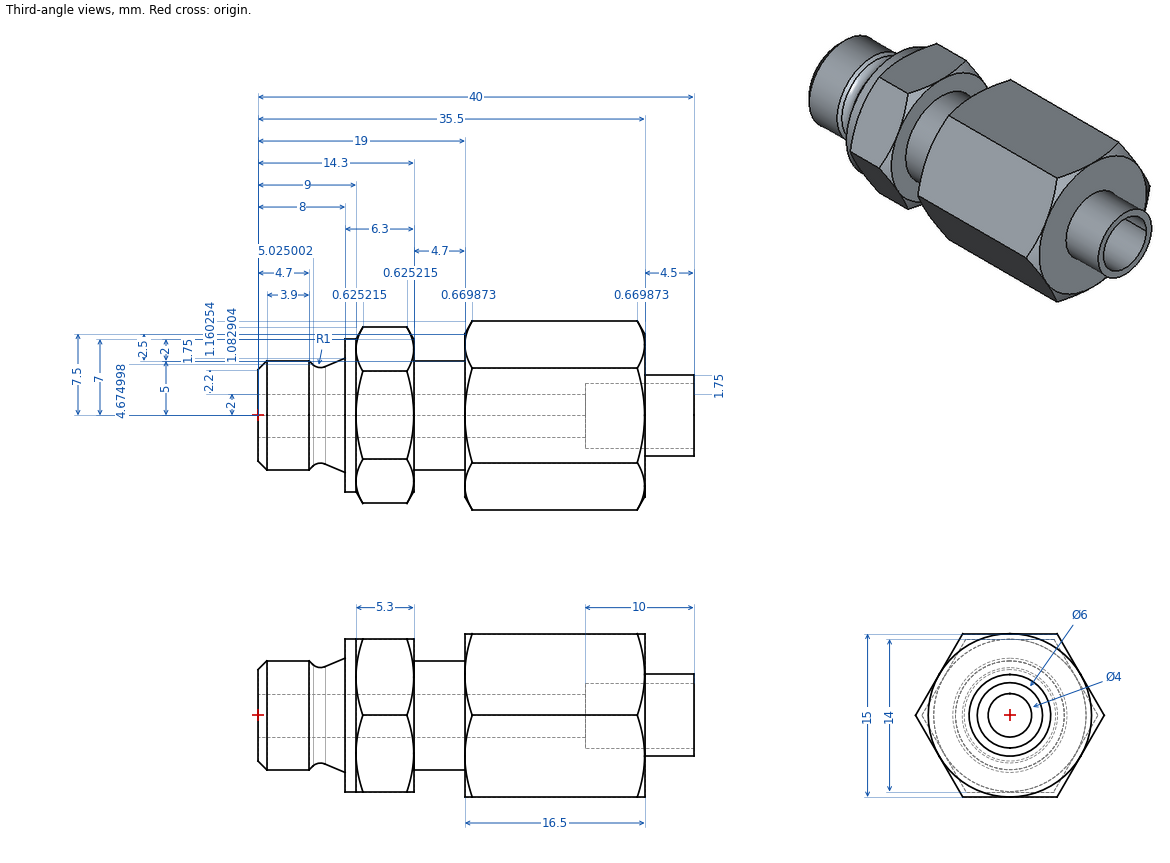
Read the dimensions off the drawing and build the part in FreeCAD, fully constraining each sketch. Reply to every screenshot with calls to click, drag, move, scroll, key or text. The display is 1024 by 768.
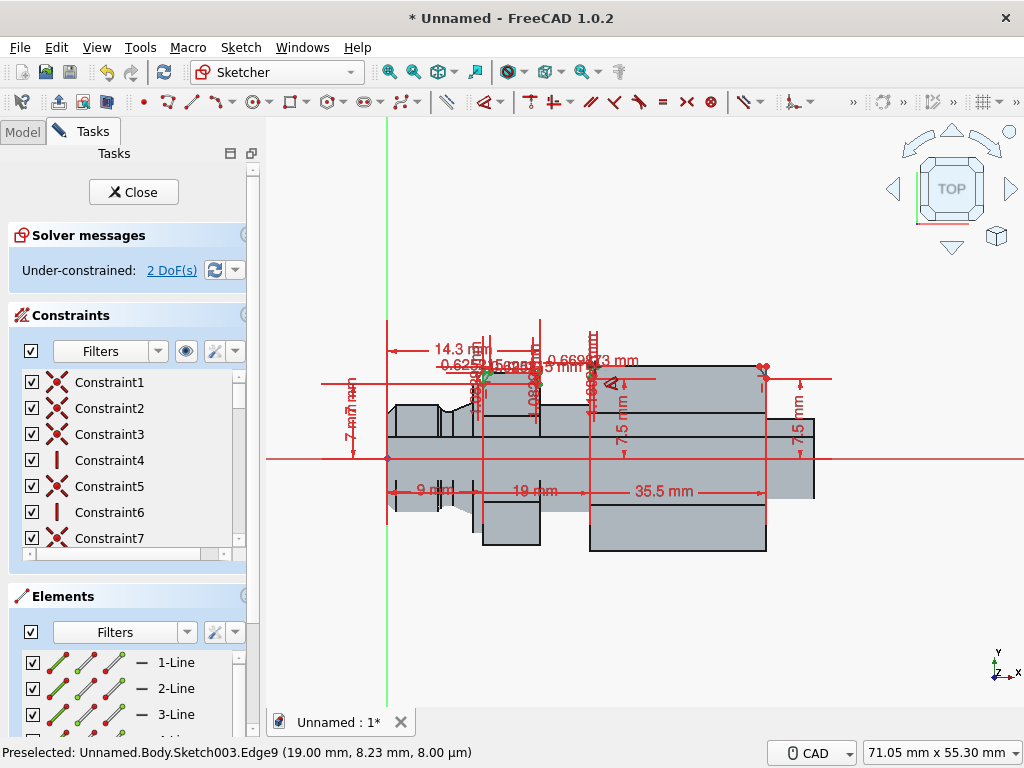
scroll(766, 375, up, 11)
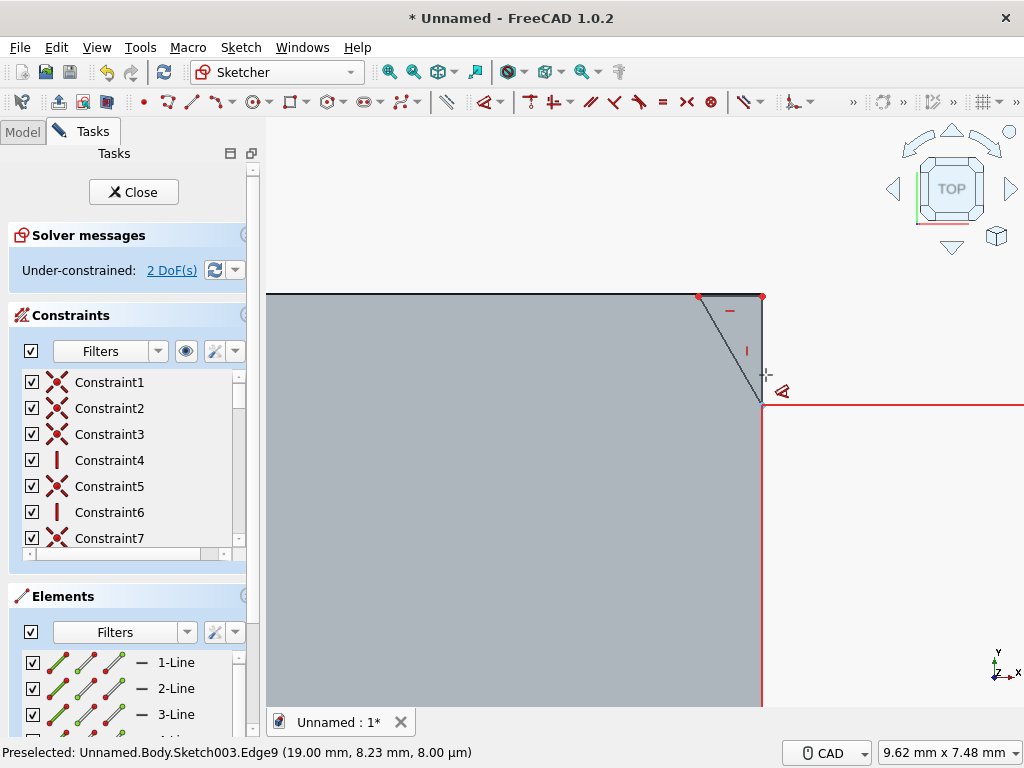
click(762, 373)
click(796, 351)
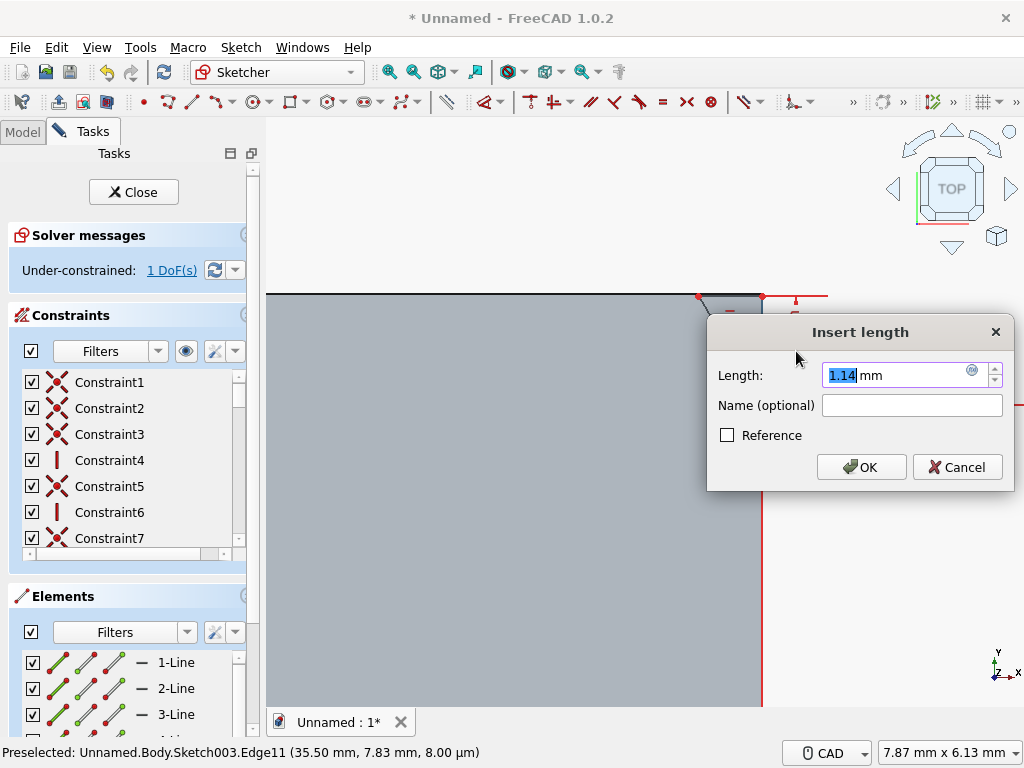
text(1.160254)
key(Return)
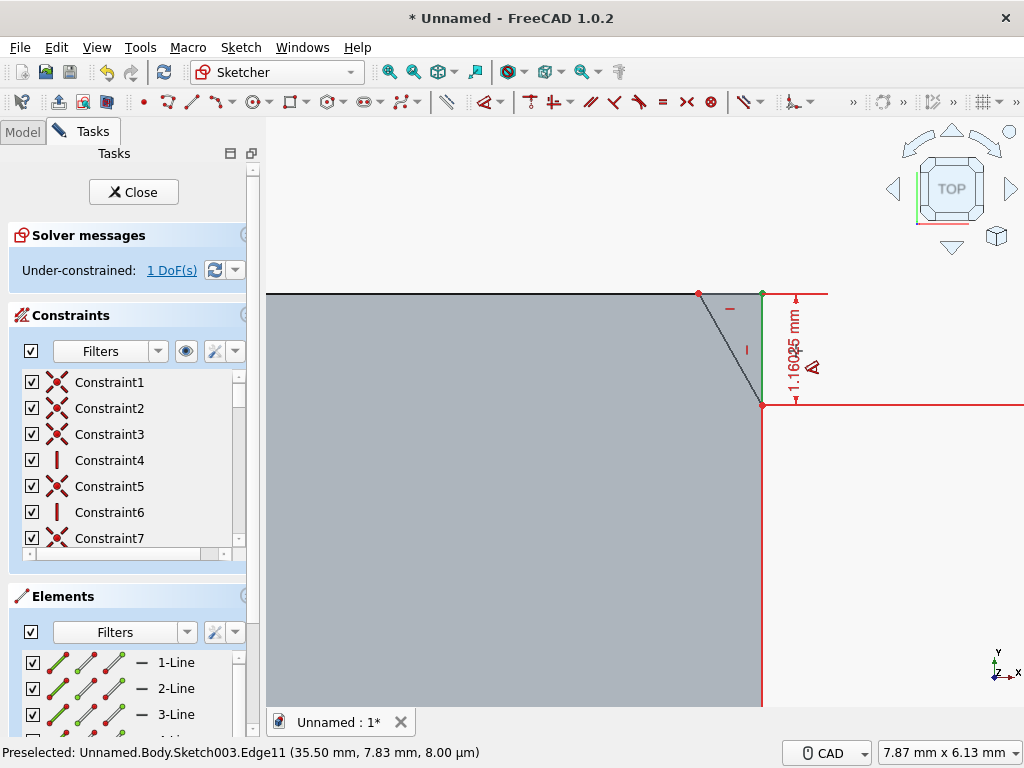
click(743, 294)
click(730, 260)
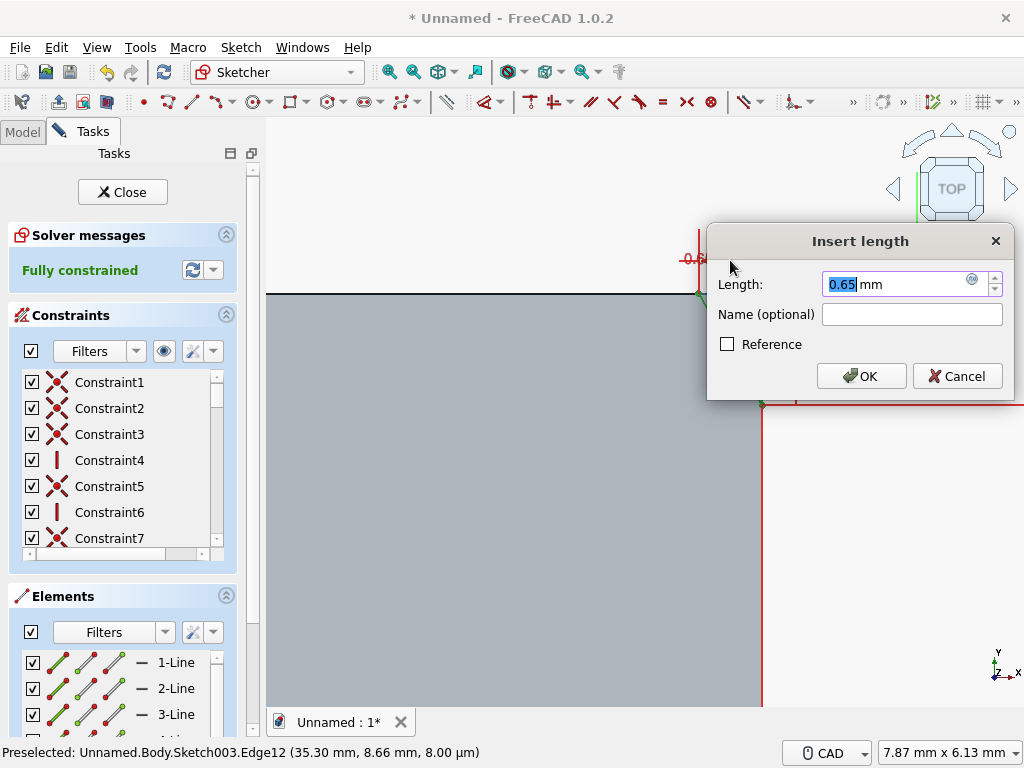
text(0.669873)
key(Return)
key(Escape)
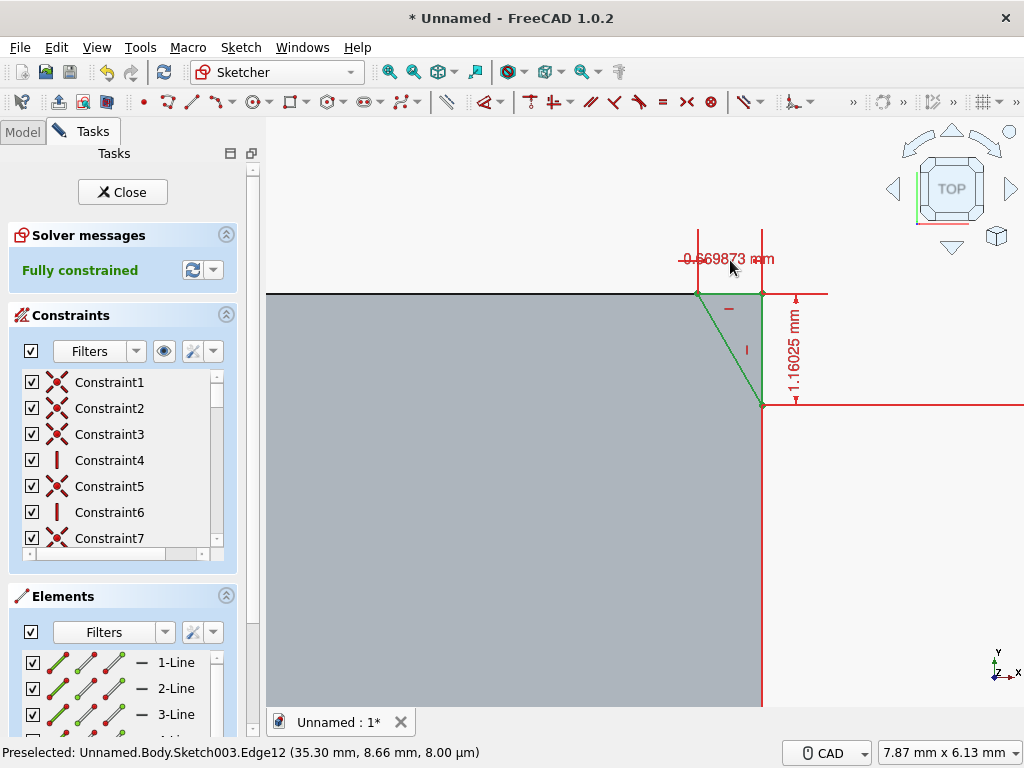
click(123, 192)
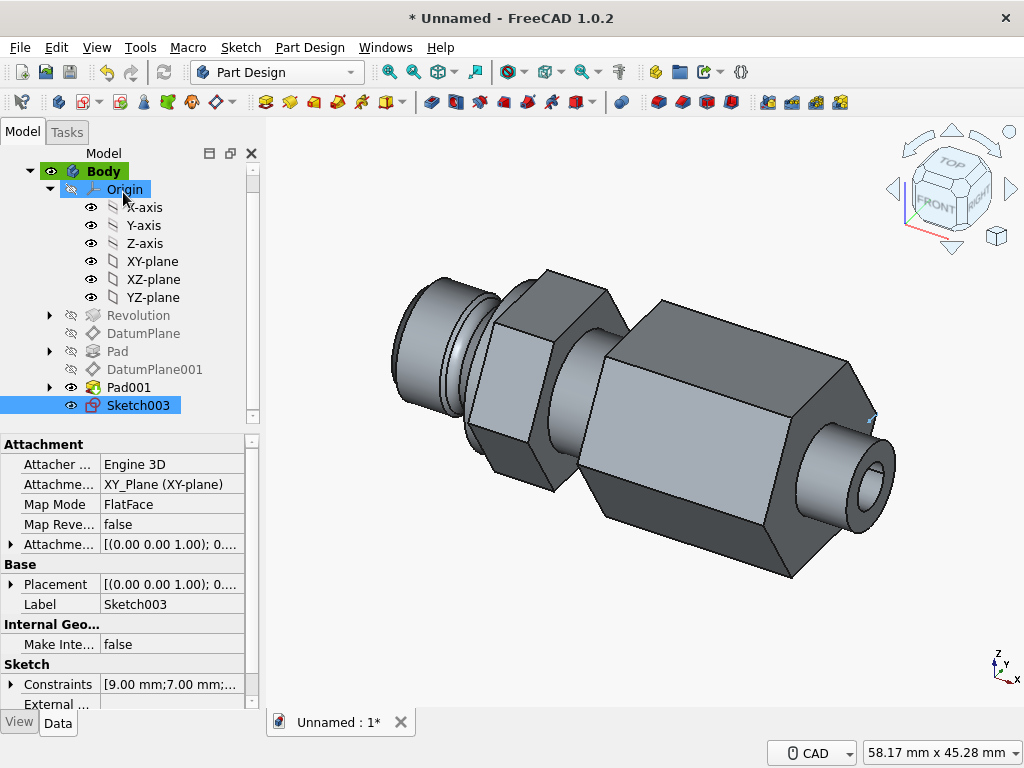
click(480, 102)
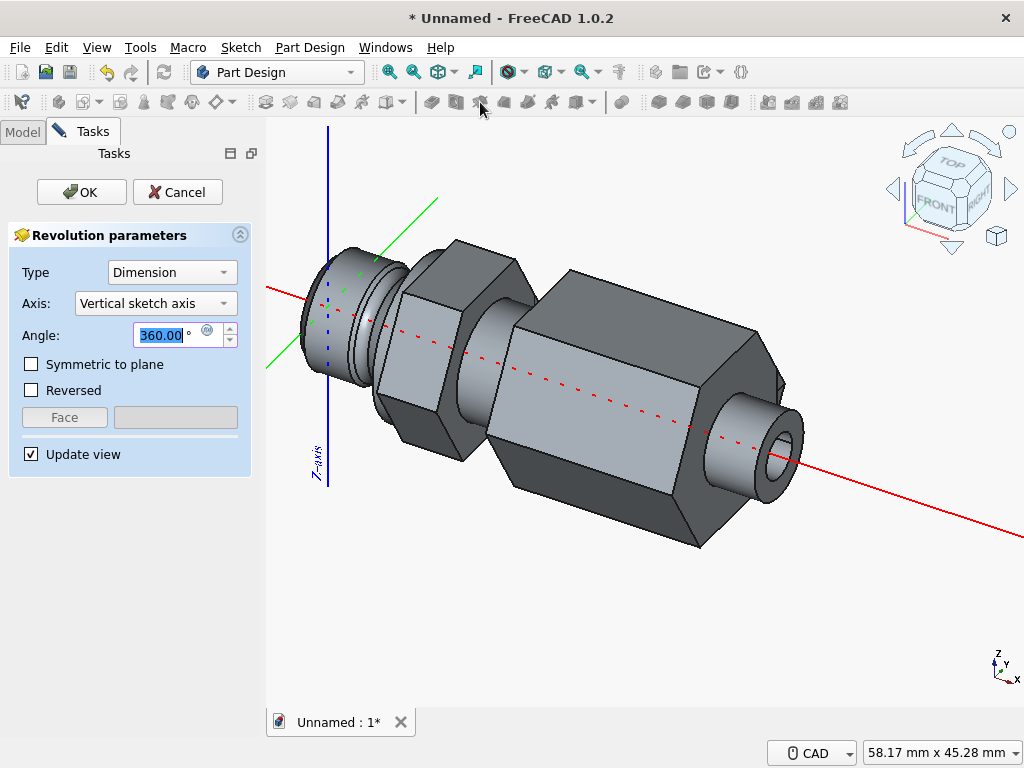
click(156, 304)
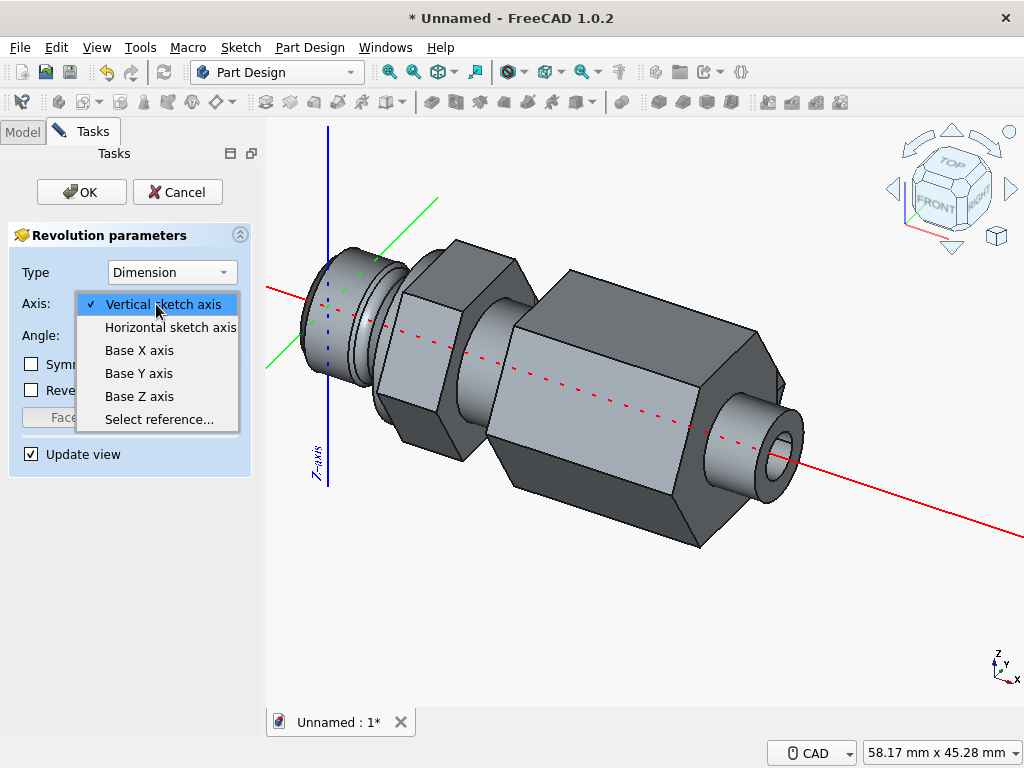
click(156, 328)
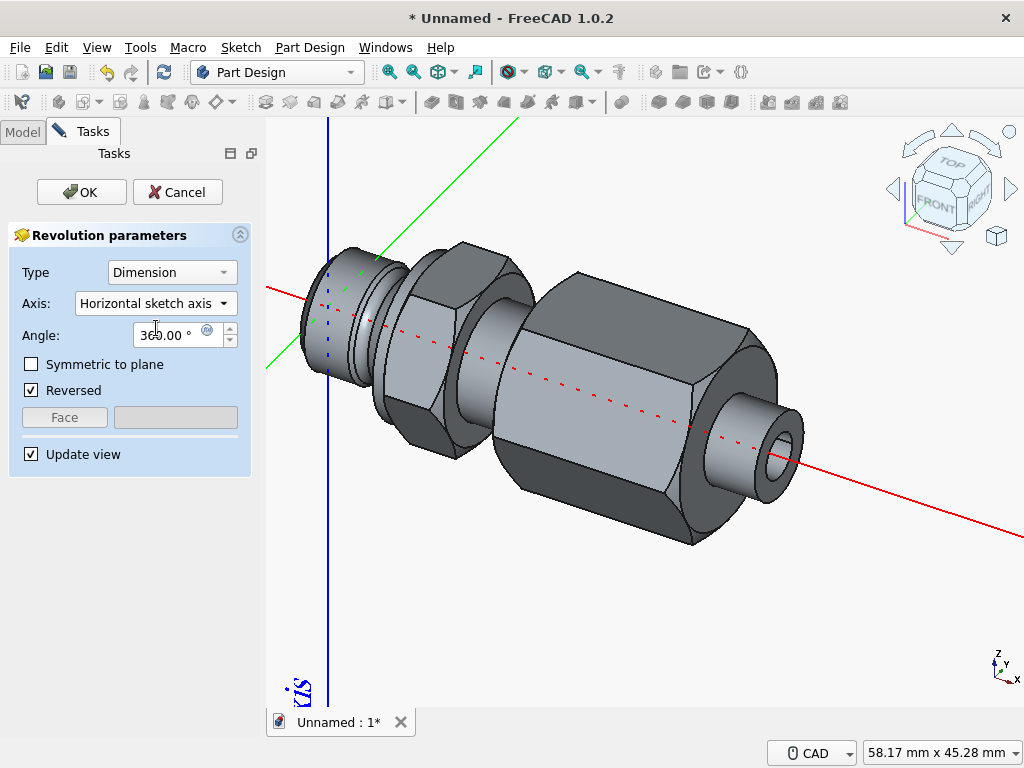
click(82, 192)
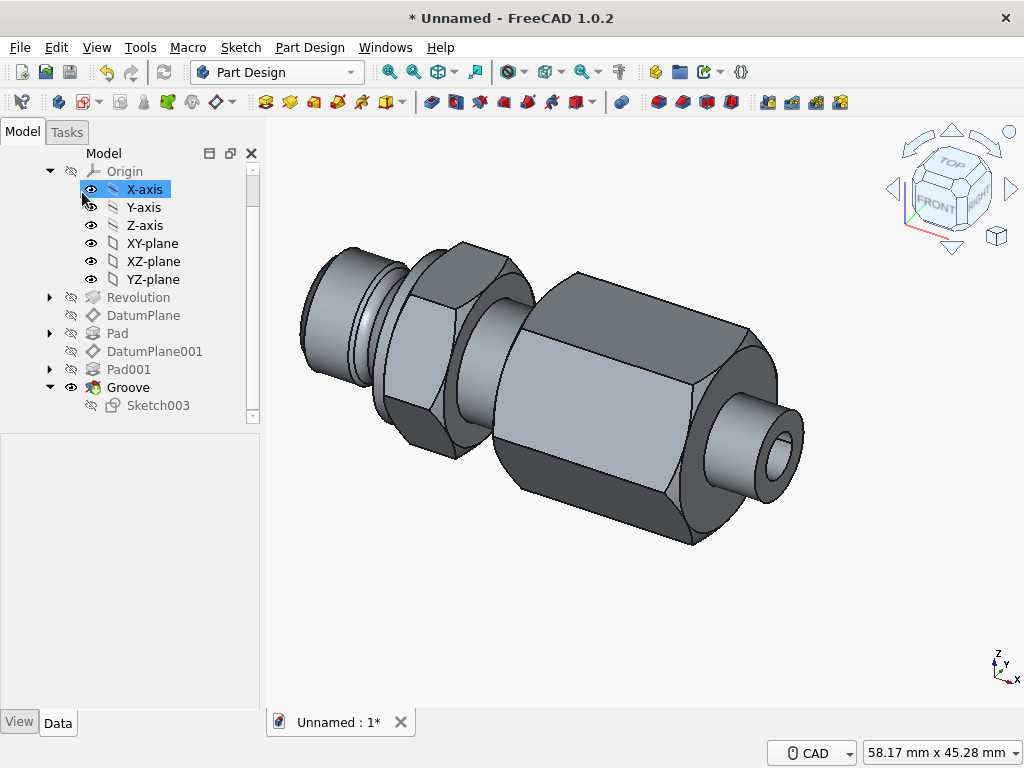
click(793, 419)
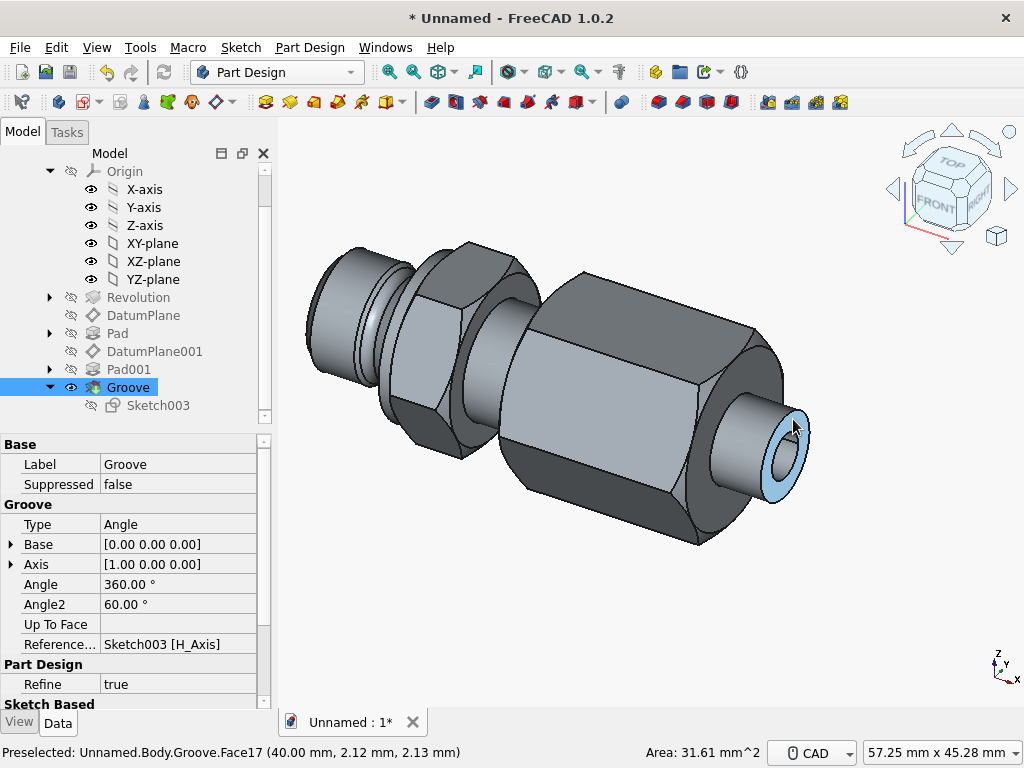
click(84, 102)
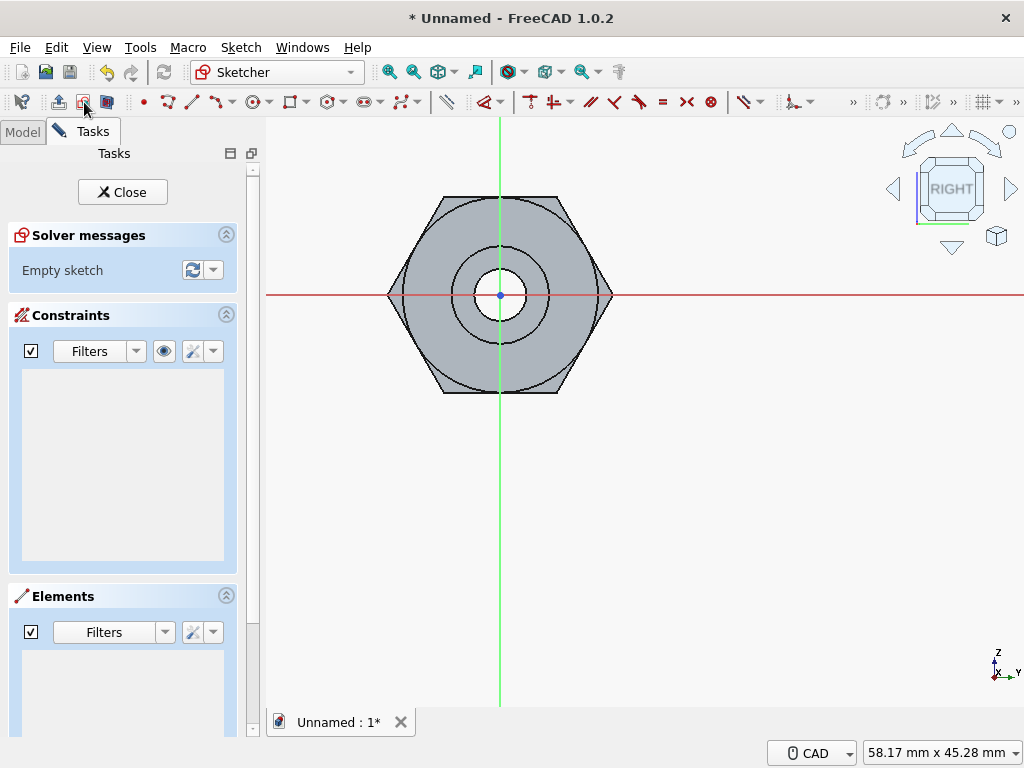
scroll(481, 265, up, 8)